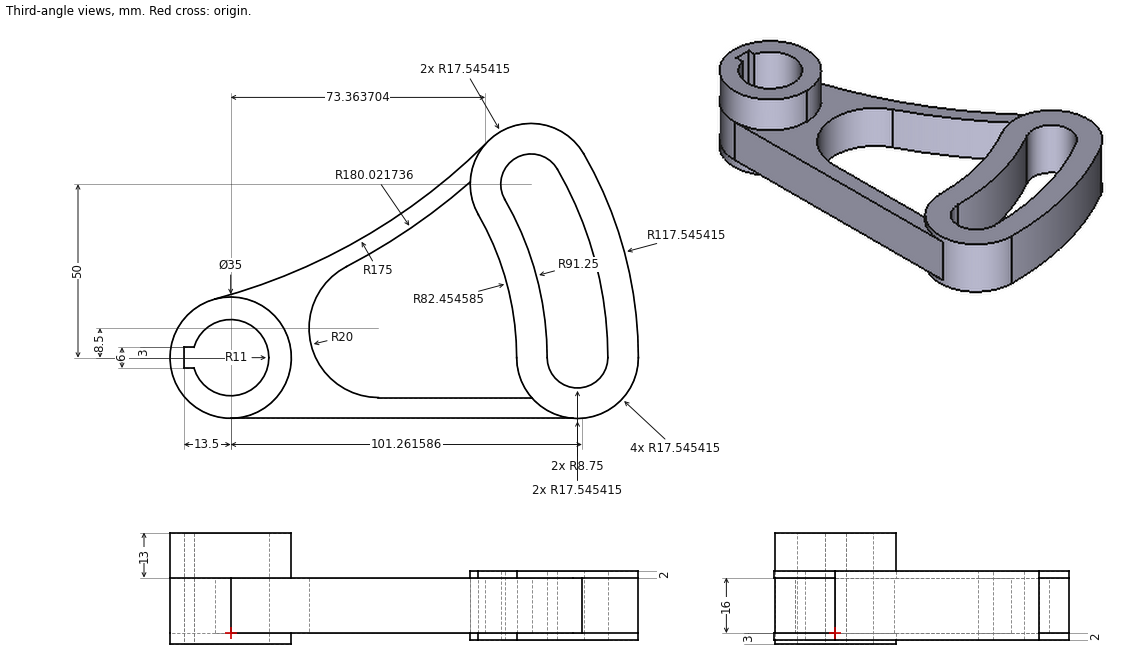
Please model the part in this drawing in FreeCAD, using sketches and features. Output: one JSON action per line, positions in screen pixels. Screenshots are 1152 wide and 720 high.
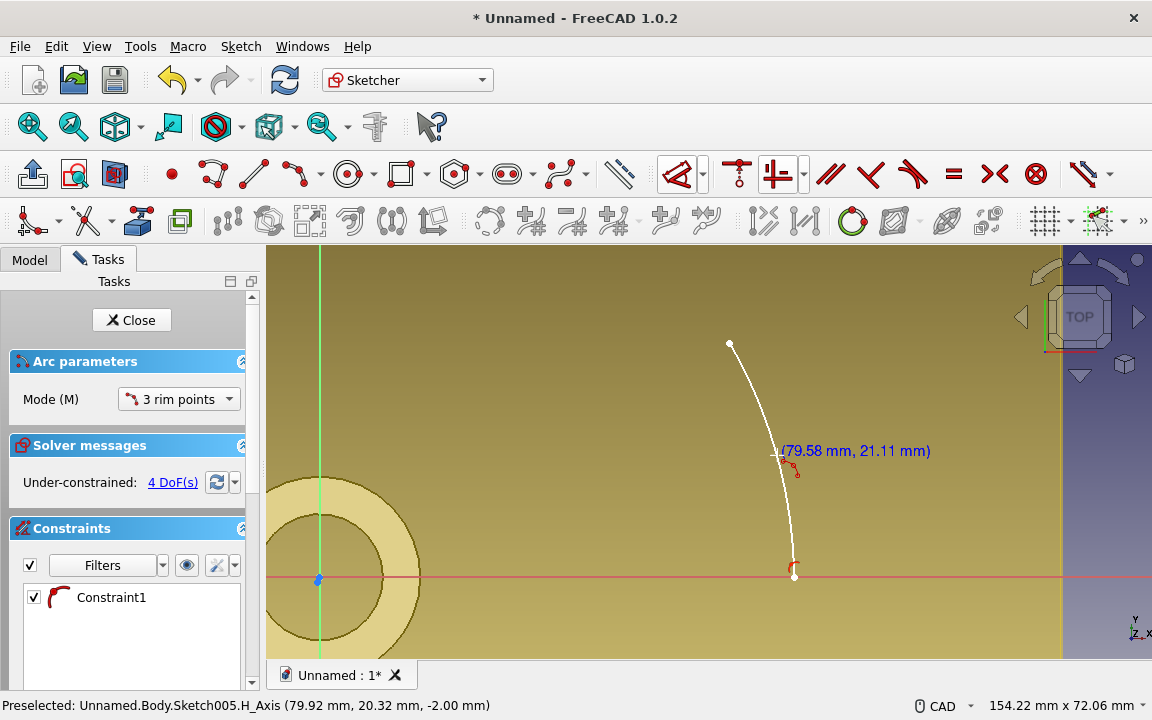
{"action": "left_click", "coordinate": [730, 343]}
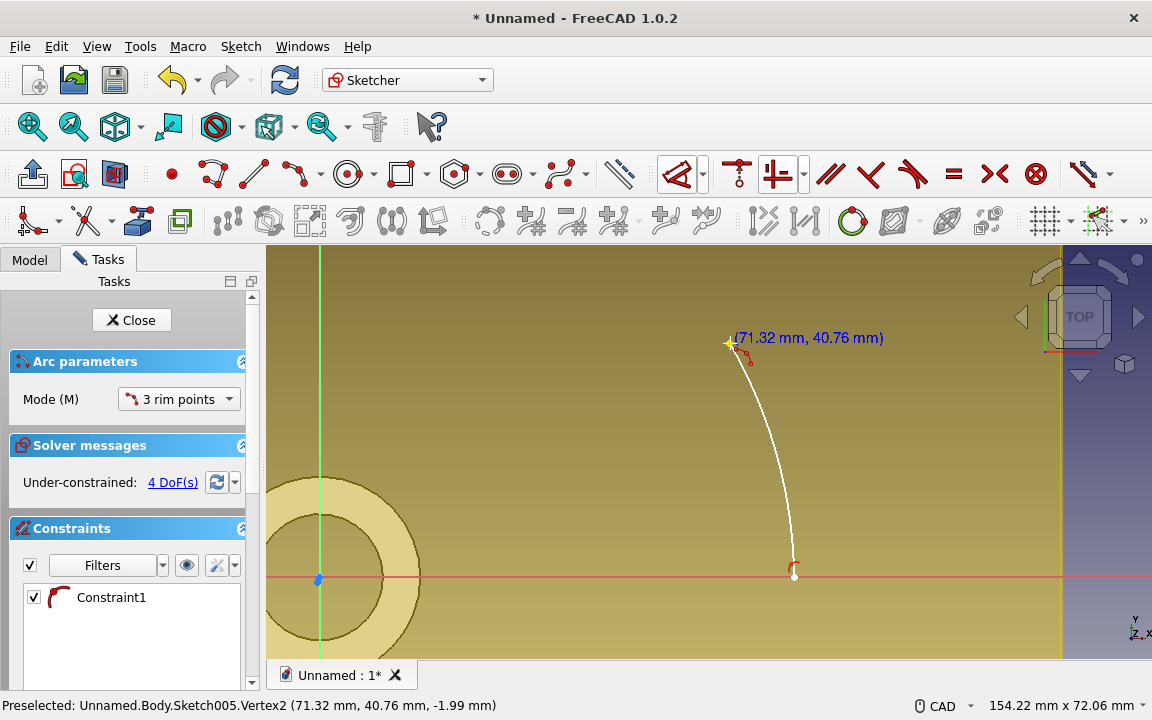
{"action": "scroll", "coordinate": [620, 466], "scroll_direction": "down", "scroll_amount": 3}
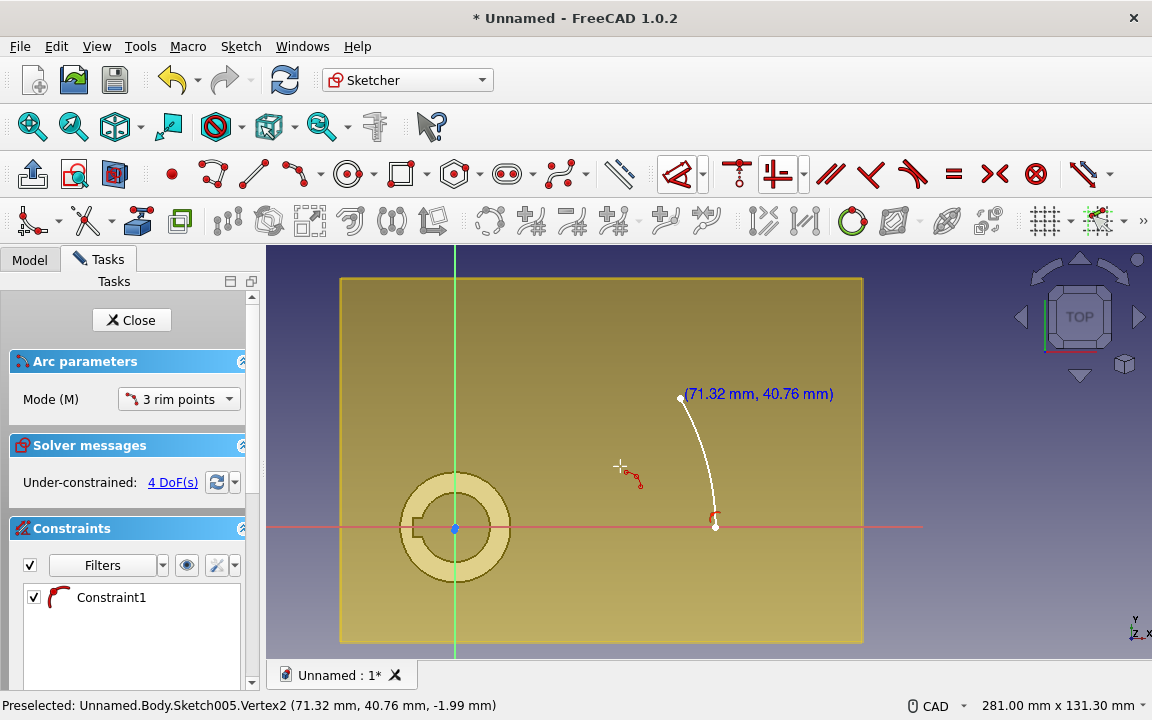
{"action": "left_click", "coordinate": [776, 342]}
{"action": "left_click", "coordinate": [701, 322]}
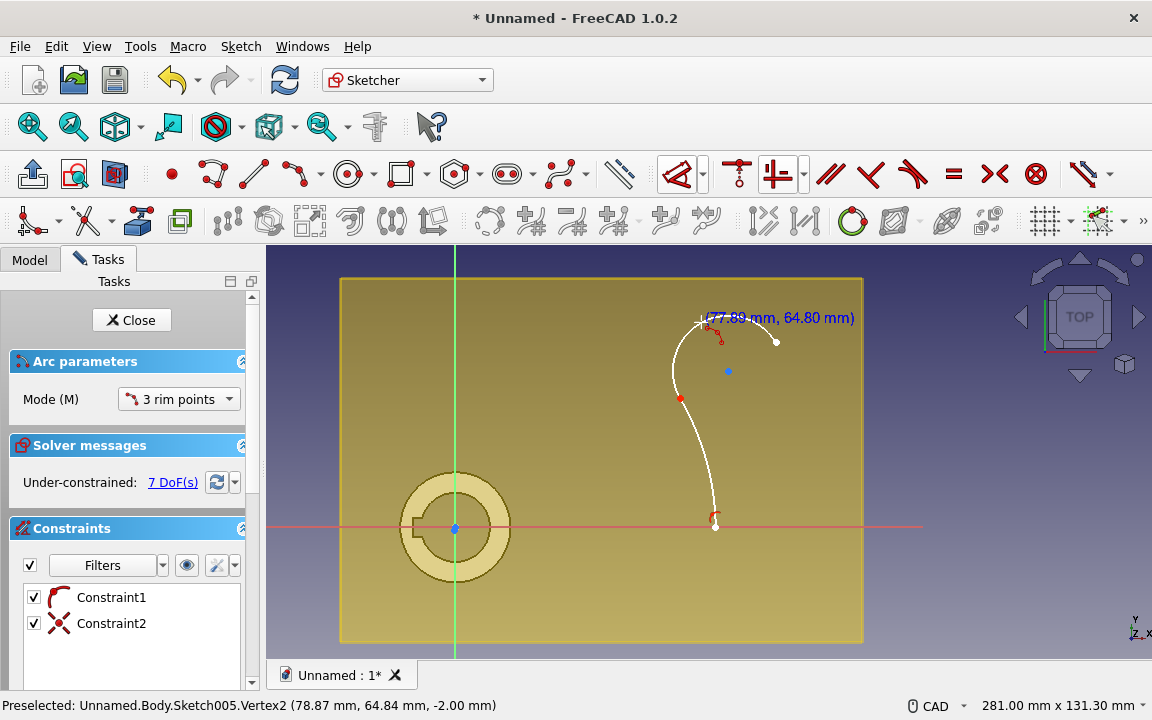
{"action": "left_click", "coordinate": [776, 343]}
{"action": "left_click", "coordinate": [826, 527]}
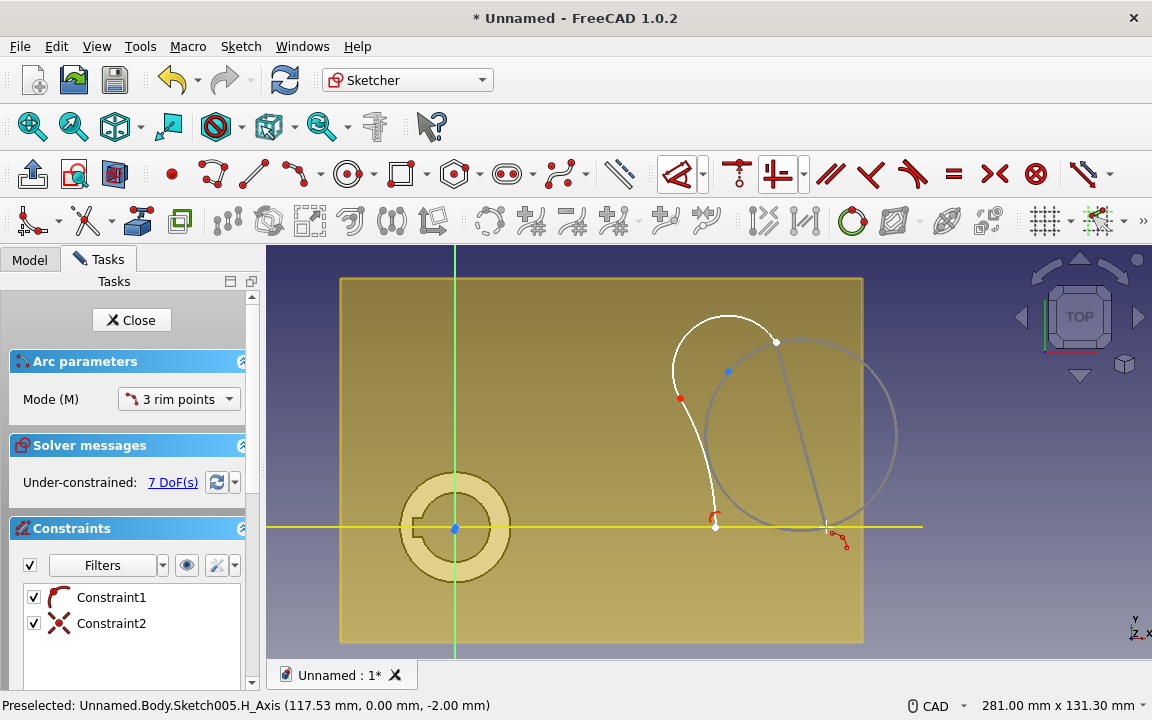
{"action": "scroll", "coordinate": [813, 431], "scroll_direction": "up", "scroll_amount": 2}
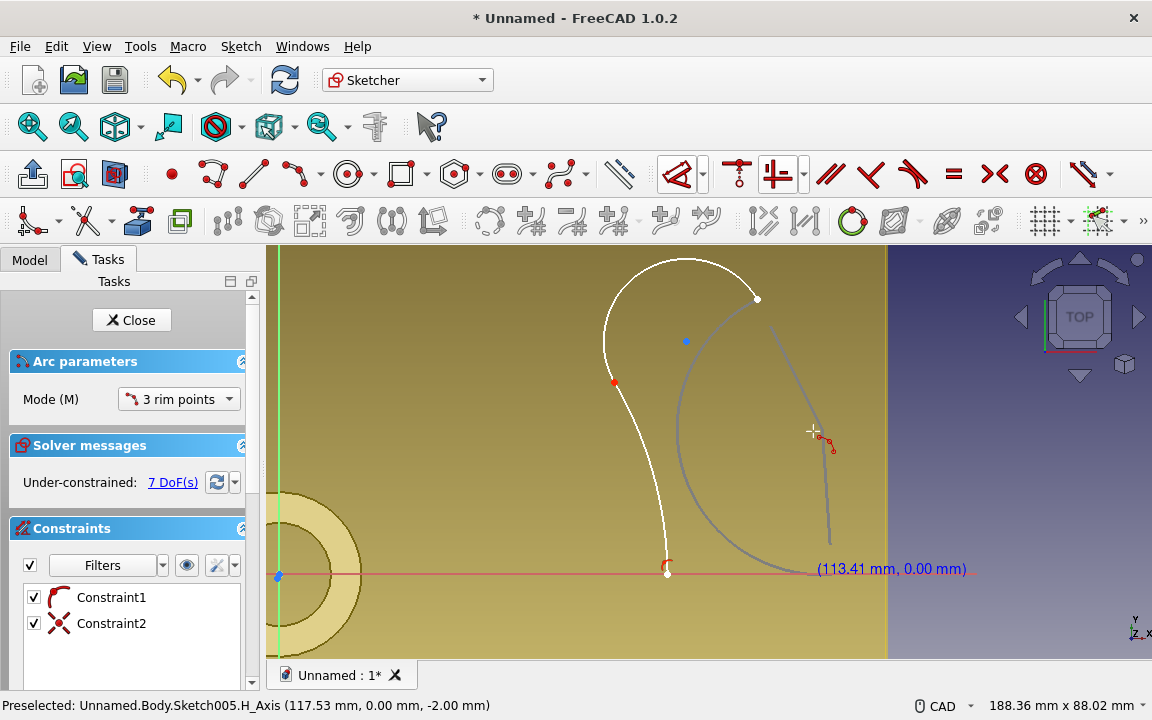
{"action": "left_click", "coordinate": [813, 431]}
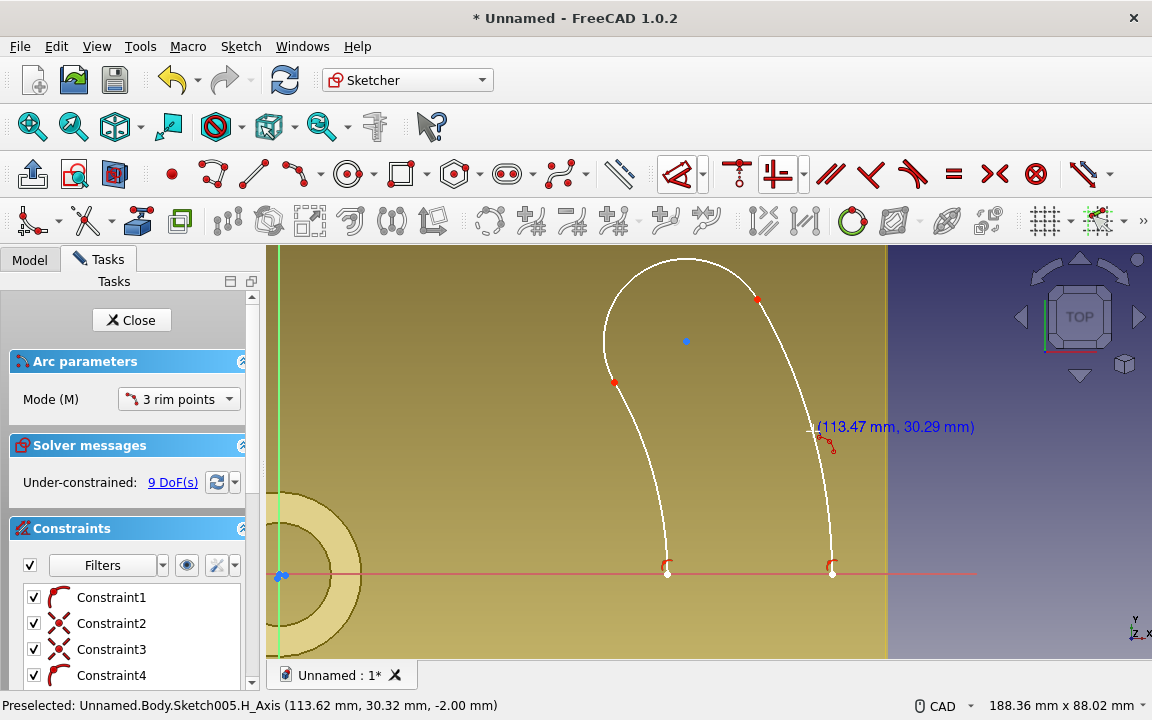
{"action": "left_click", "coordinate": [832, 574]}
{"action": "left_click", "coordinate": [668, 574]}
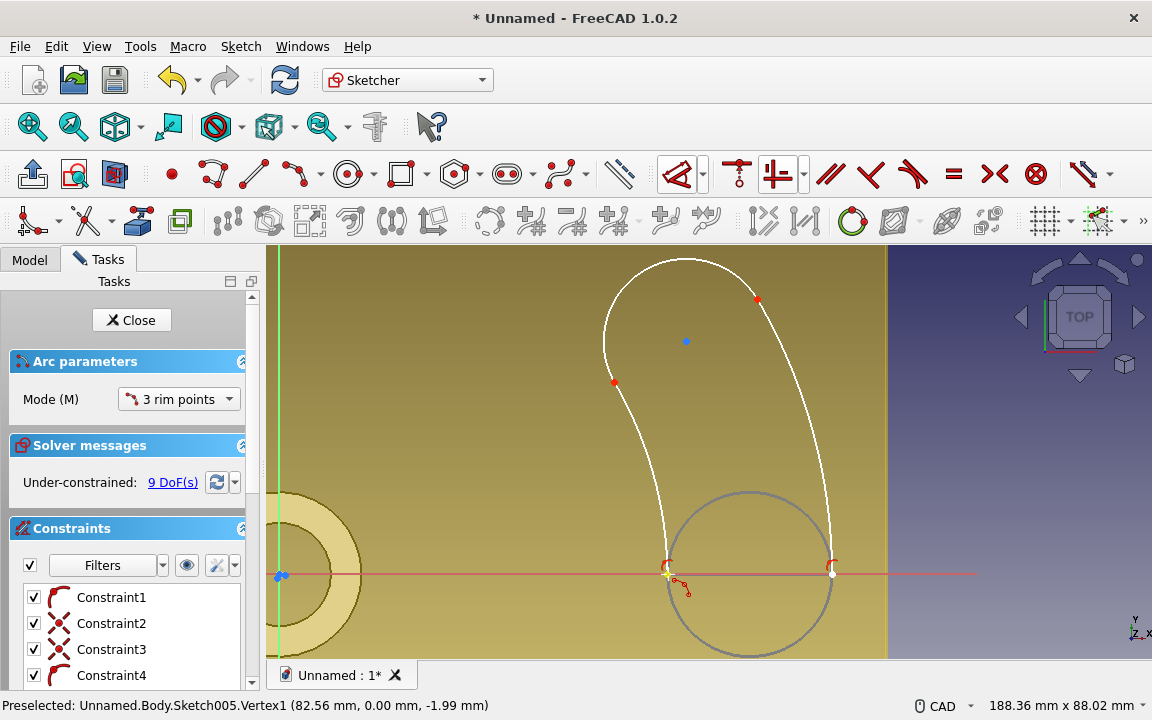
{"action": "scroll", "coordinate": [813, 431], "scroll_direction": "down", "scroll_amount": 2}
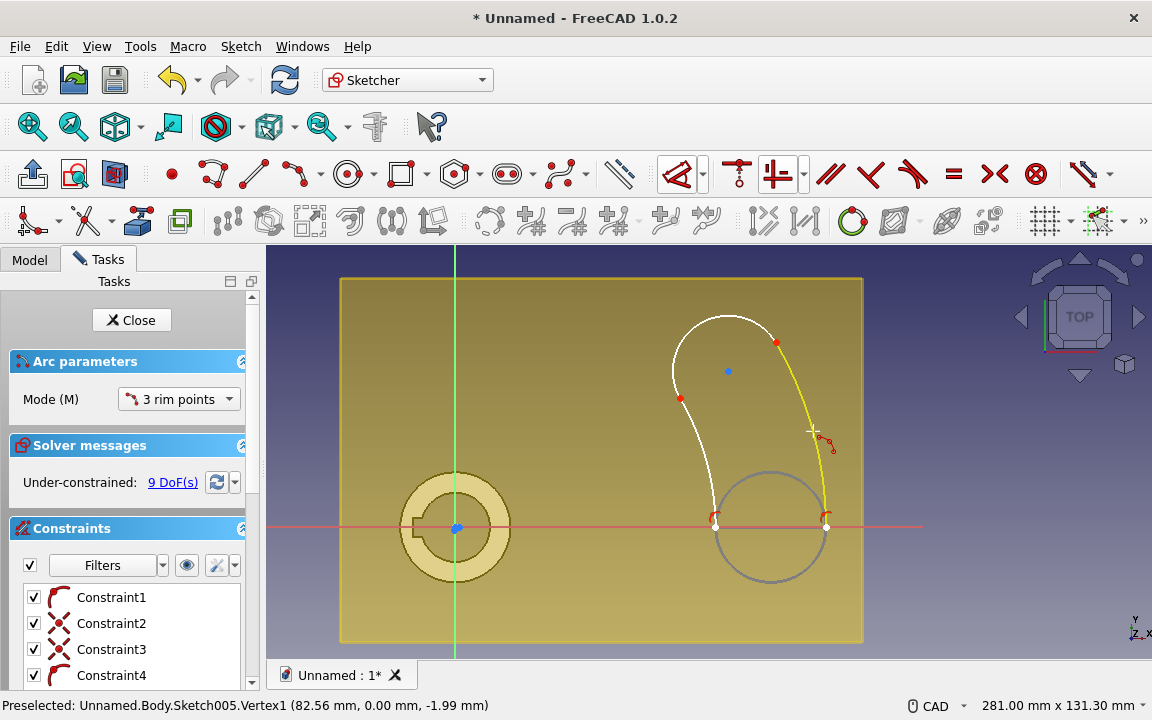
{"action": "left_click", "coordinate": [771, 583]}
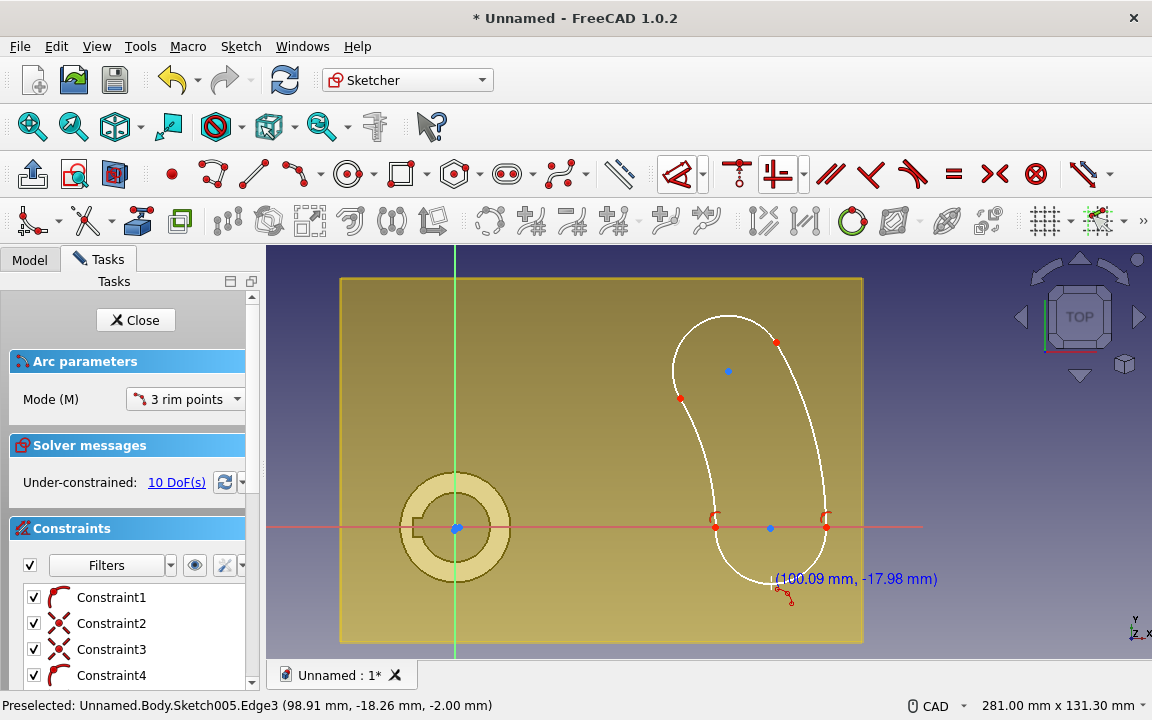
{"action": "left_click", "coordinate": [705, 383]}
{"action": "left_click", "coordinate": [743, 527]}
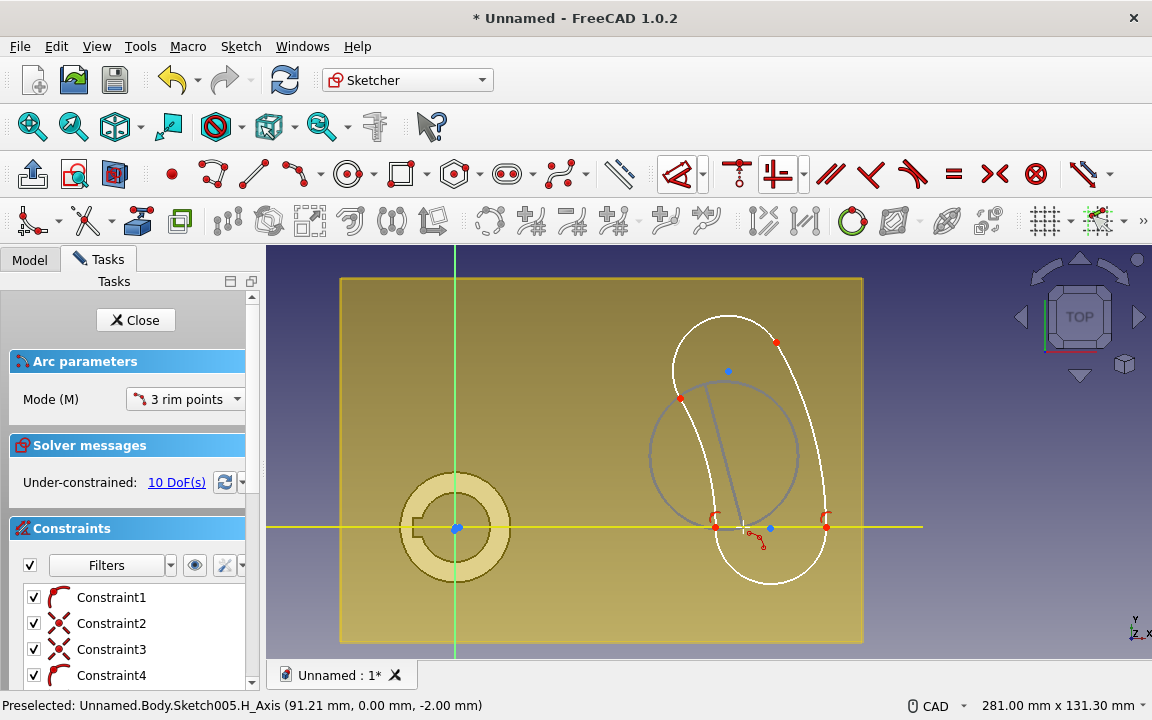
{"action": "scroll", "coordinate": [733, 453], "scroll_direction": "up", "scroll_amount": 3}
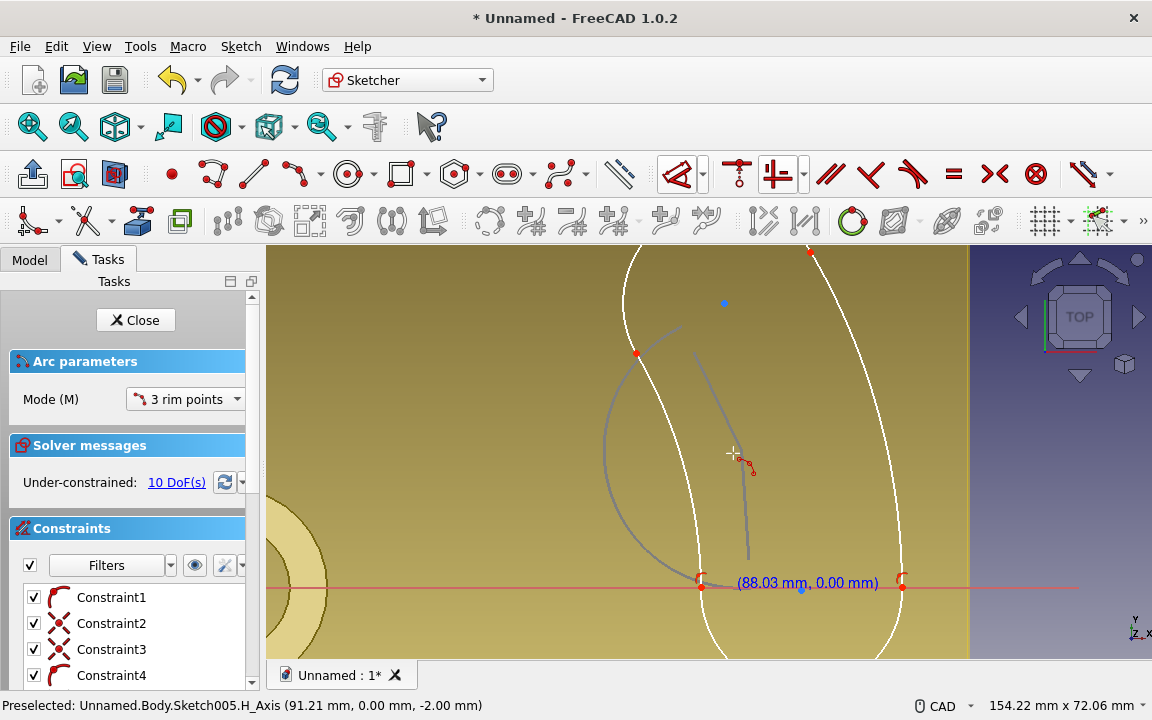
{"action": "left_click", "coordinate": [733, 452]}